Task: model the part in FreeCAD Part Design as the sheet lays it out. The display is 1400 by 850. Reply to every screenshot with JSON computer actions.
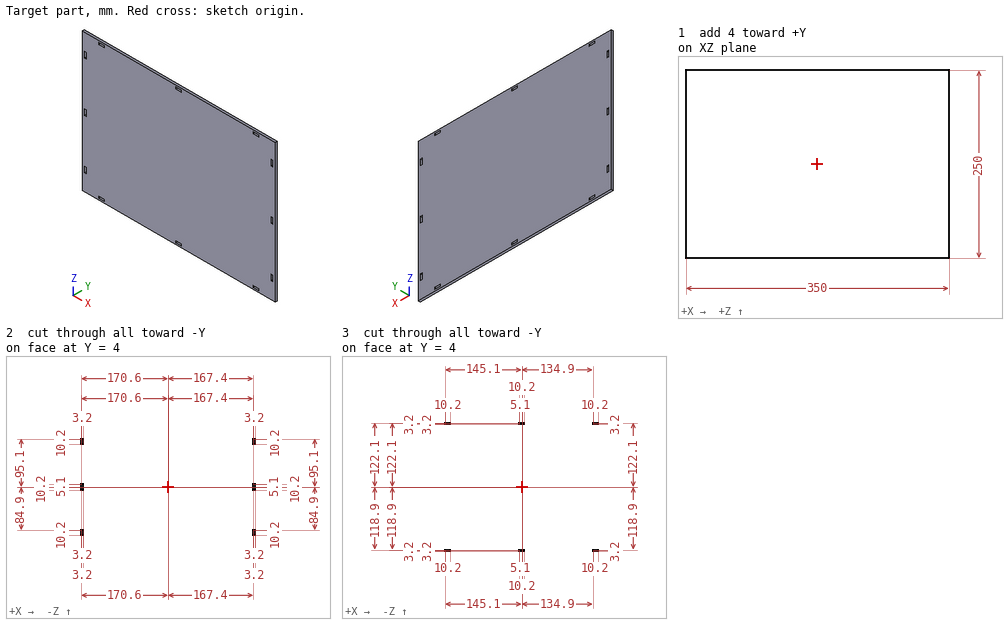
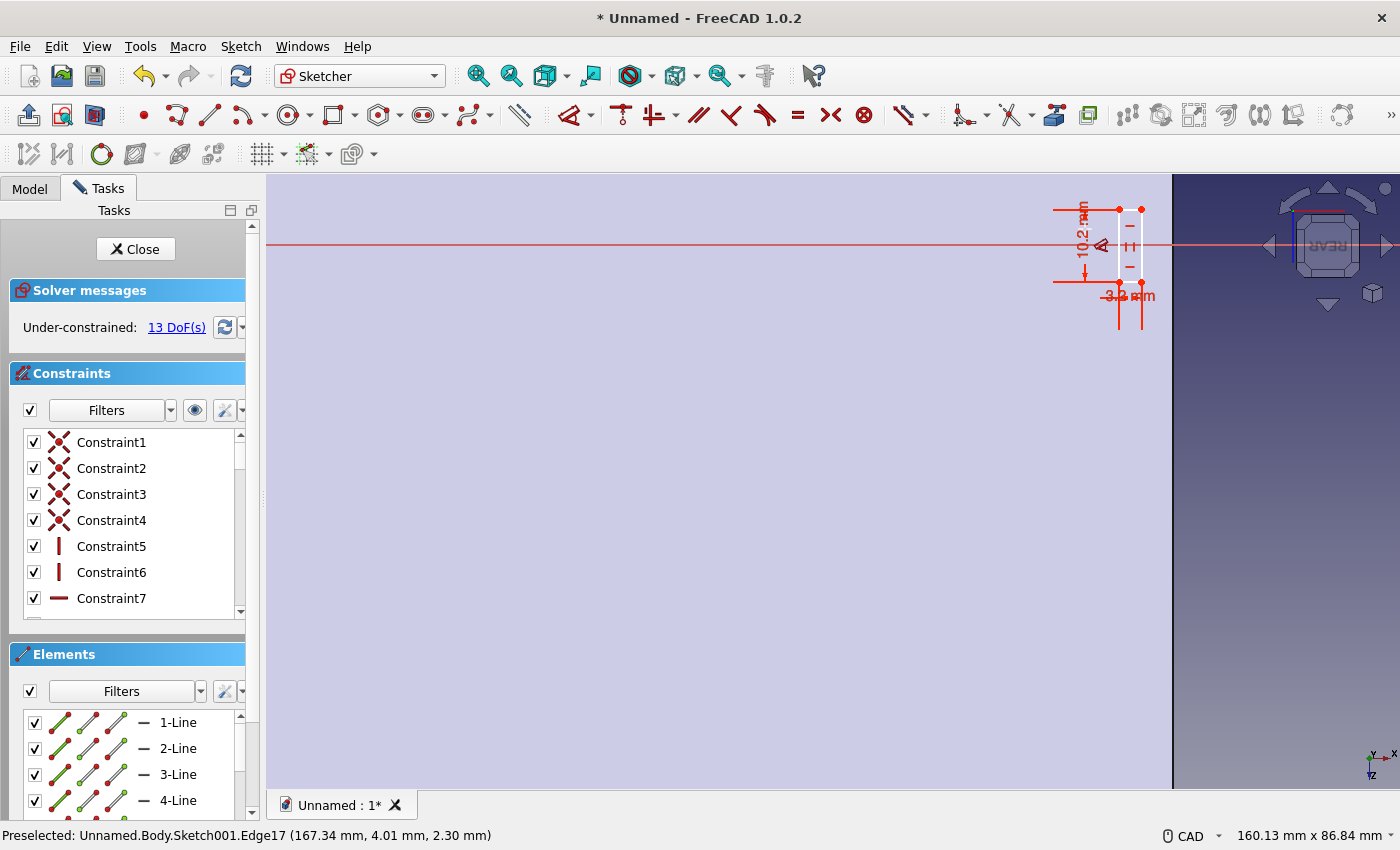
{"action": "scroll", "coordinate": [1122, 584], "scroll_direction": "down", "scroll_amount": 6}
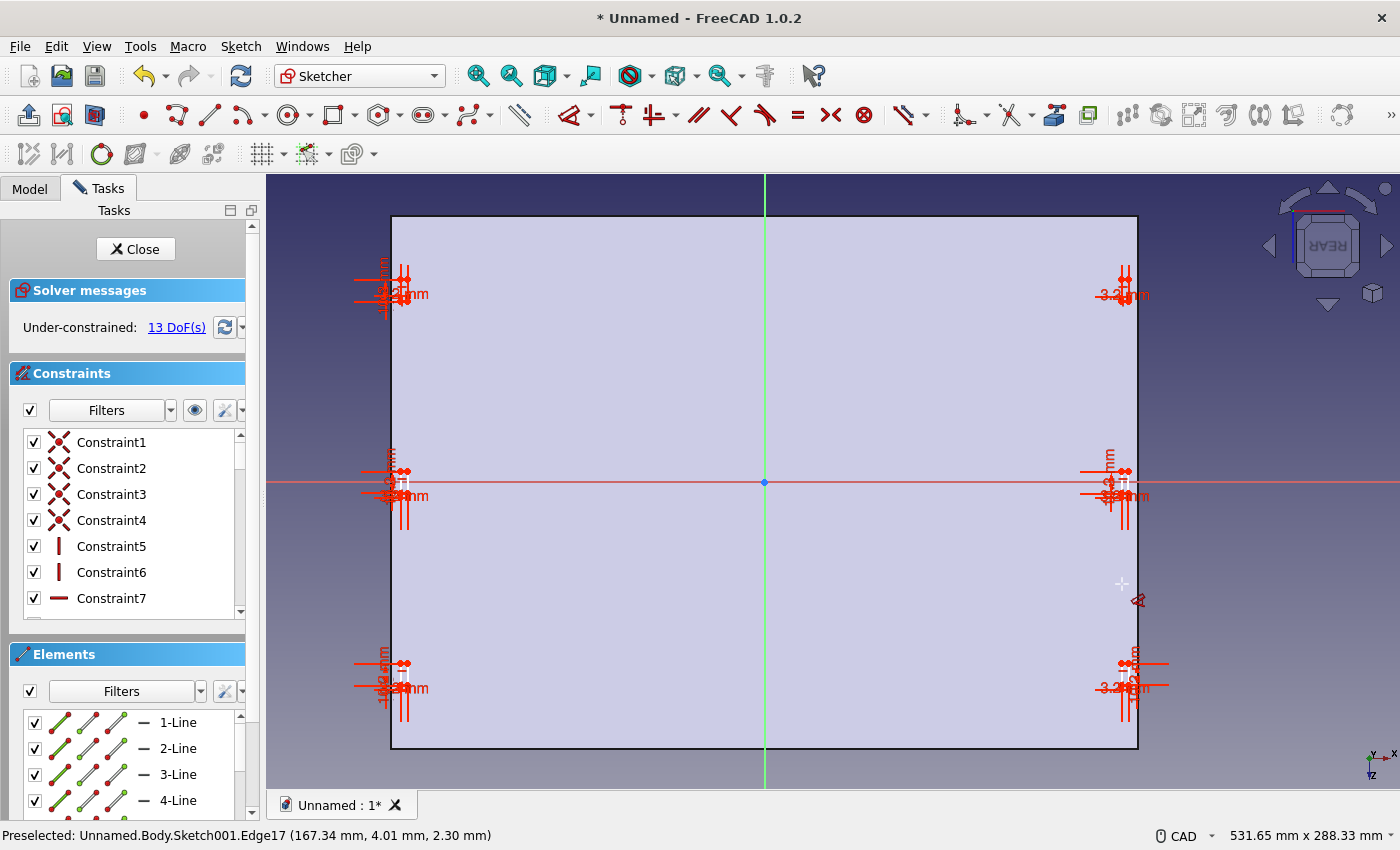
{"action": "scroll", "coordinate": [1122, 286], "scroll_direction": "up", "scroll_amount": 4}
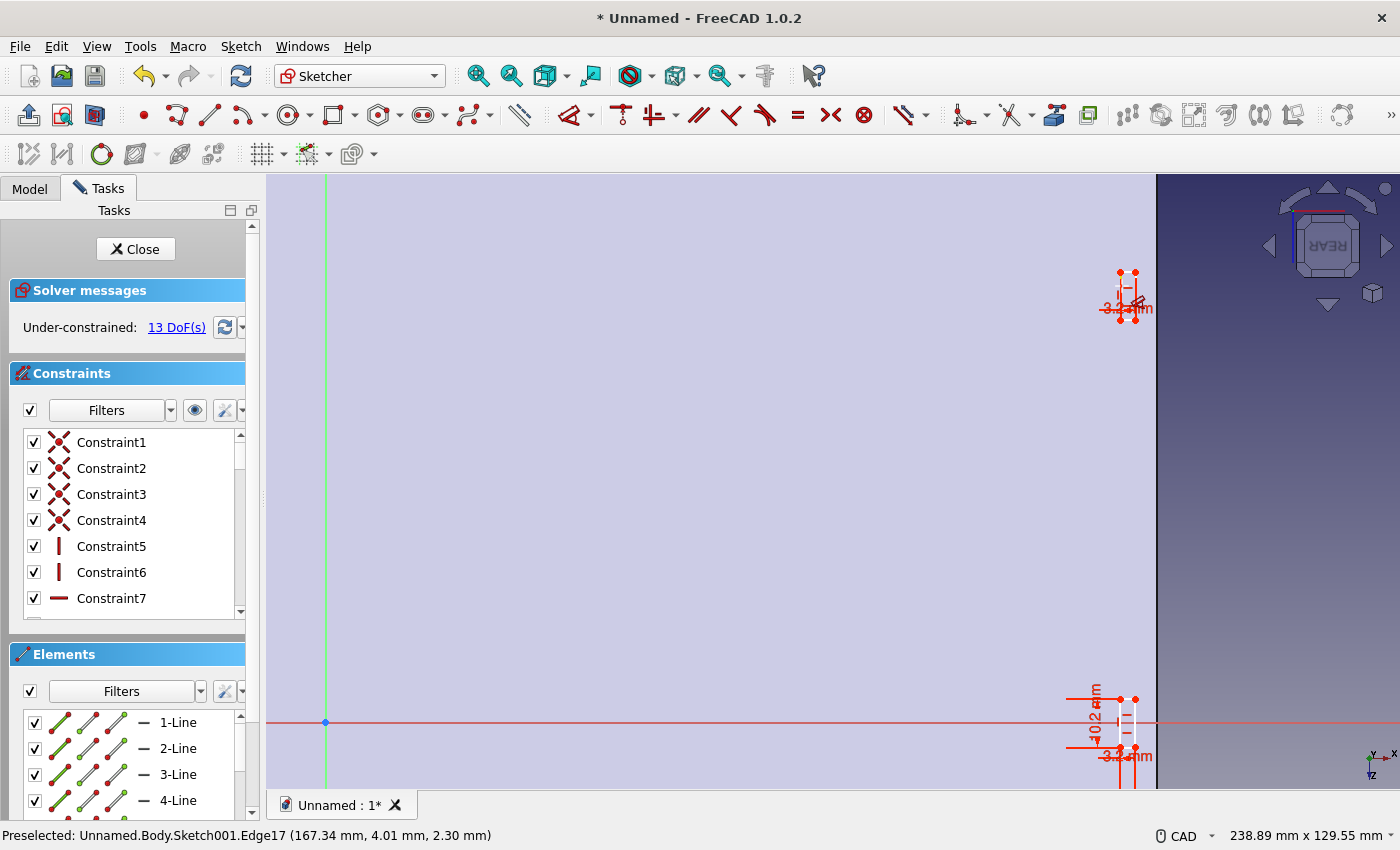
{"action": "left_click", "coordinate": [1121, 287]}
{"action": "left_click", "coordinate": [1155, 285]}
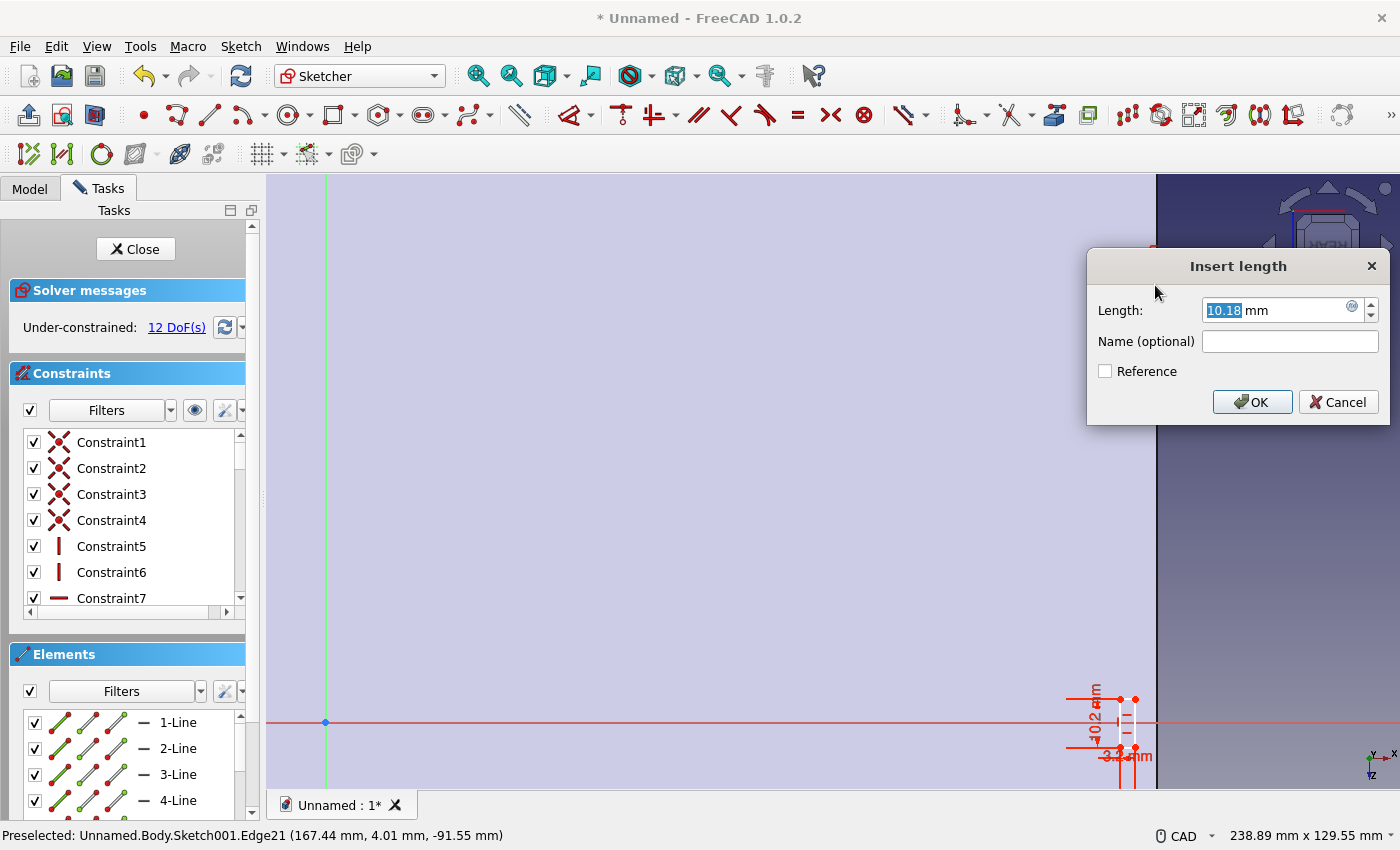
{"action": "type", "text": "10.2"}
{"action": "key", "text": "Return"}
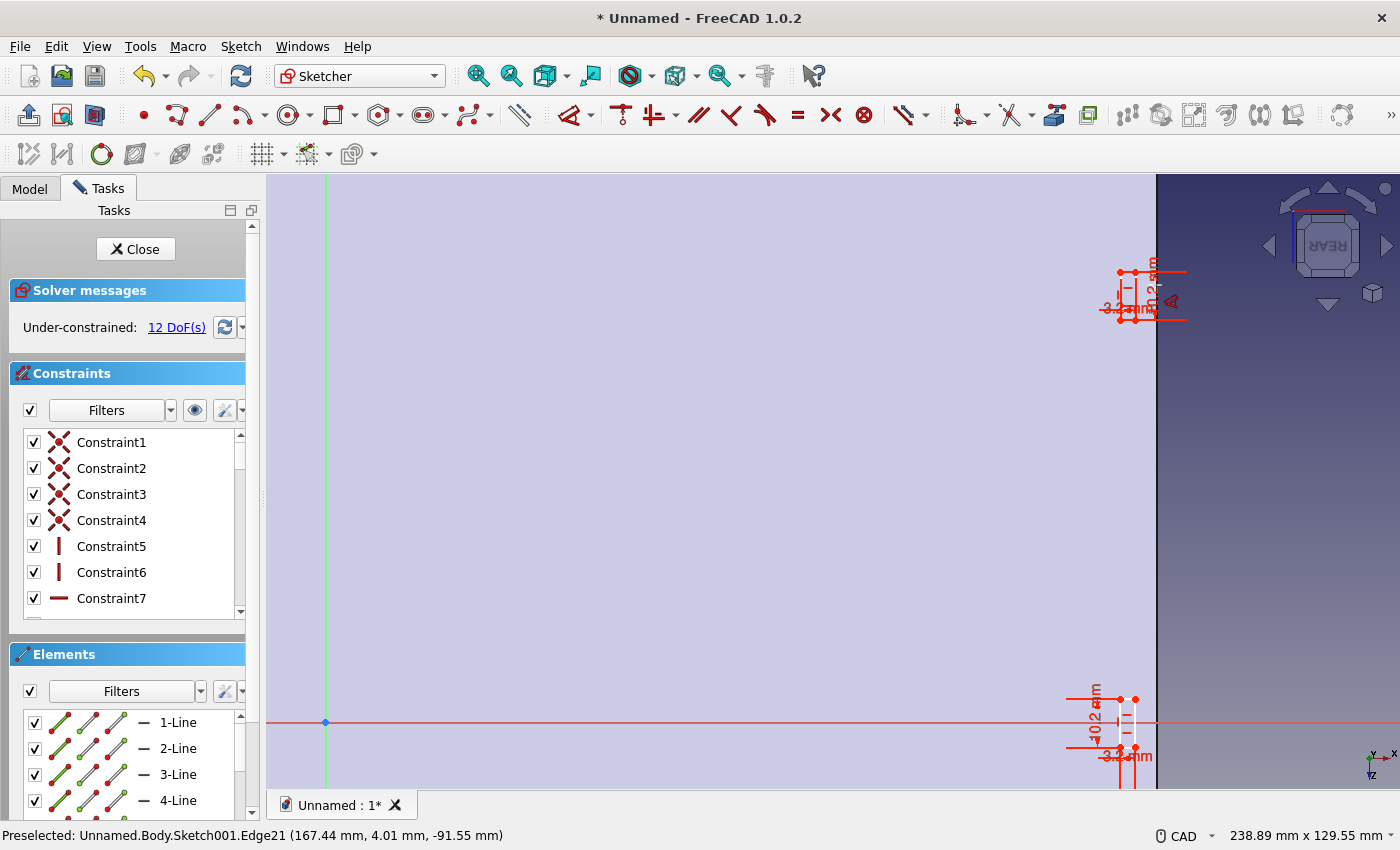
{"action": "scroll", "coordinate": [1122, 285], "scroll_direction": "down", "scroll_amount": 4}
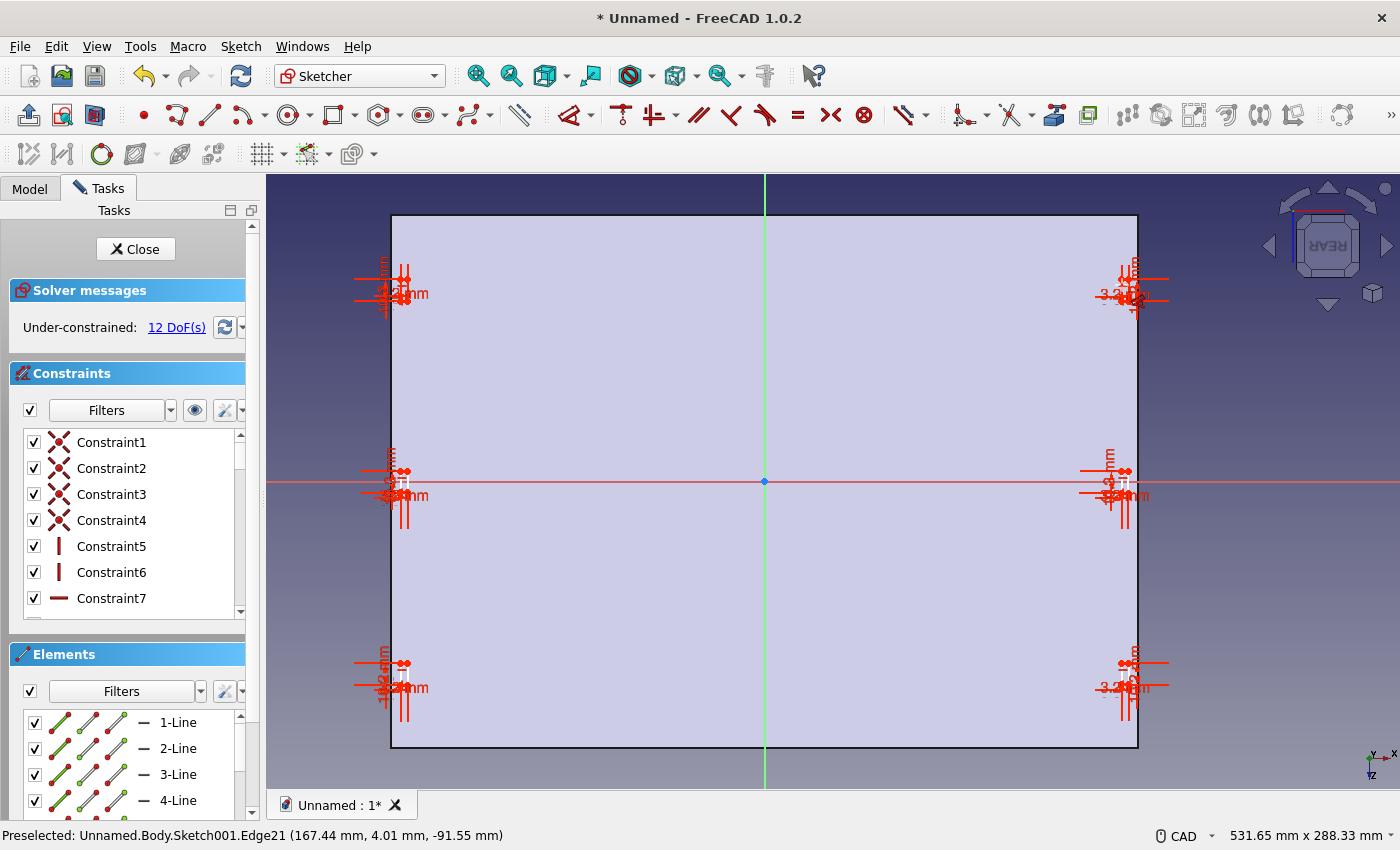
{"action": "scroll", "coordinate": [401, 471], "scroll_direction": "up", "scroll_amount": 7}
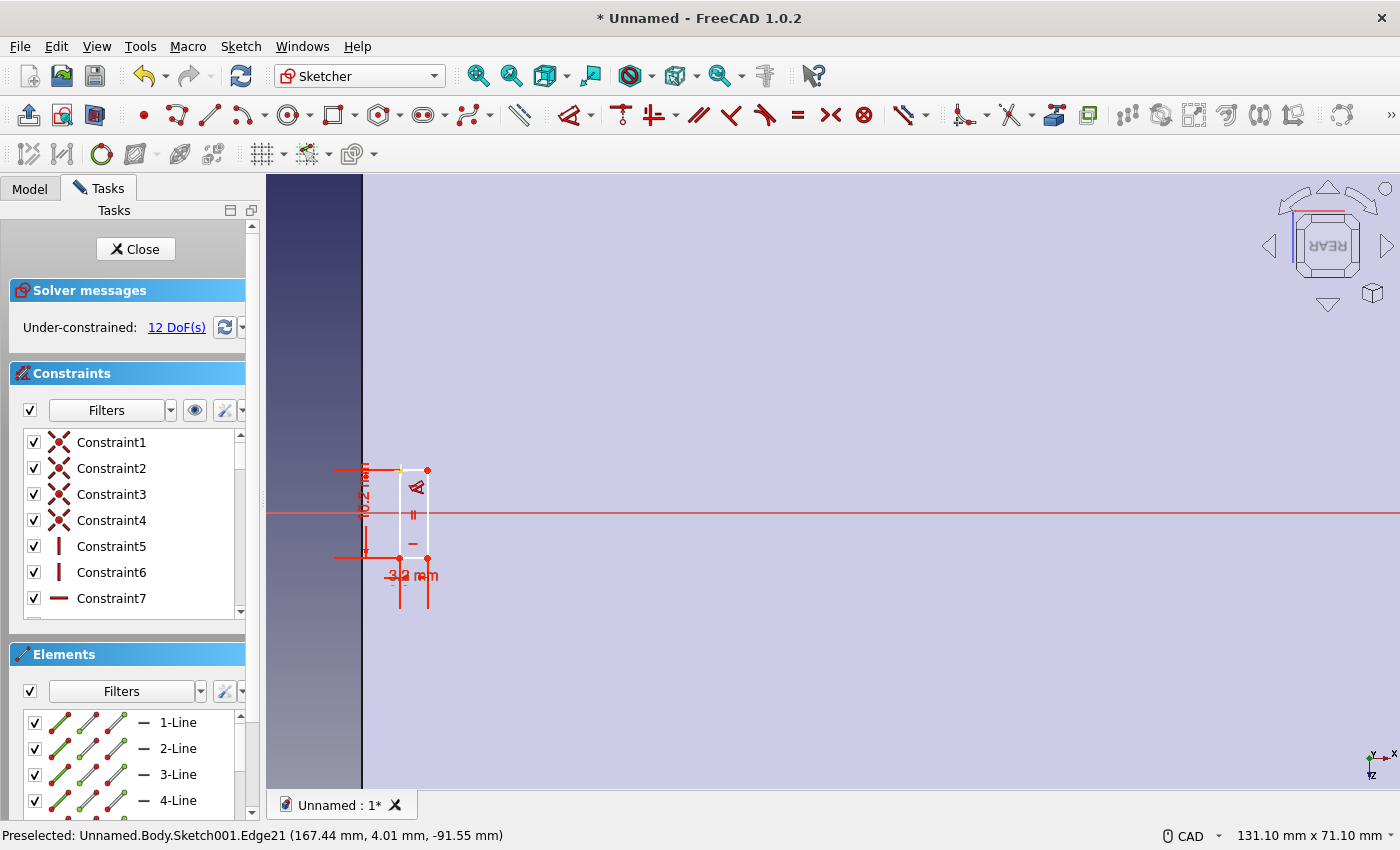
{"action": "left_click", "coordinate": [400, 470]}
{"action": "left_click", "coordinate": [366, 501]}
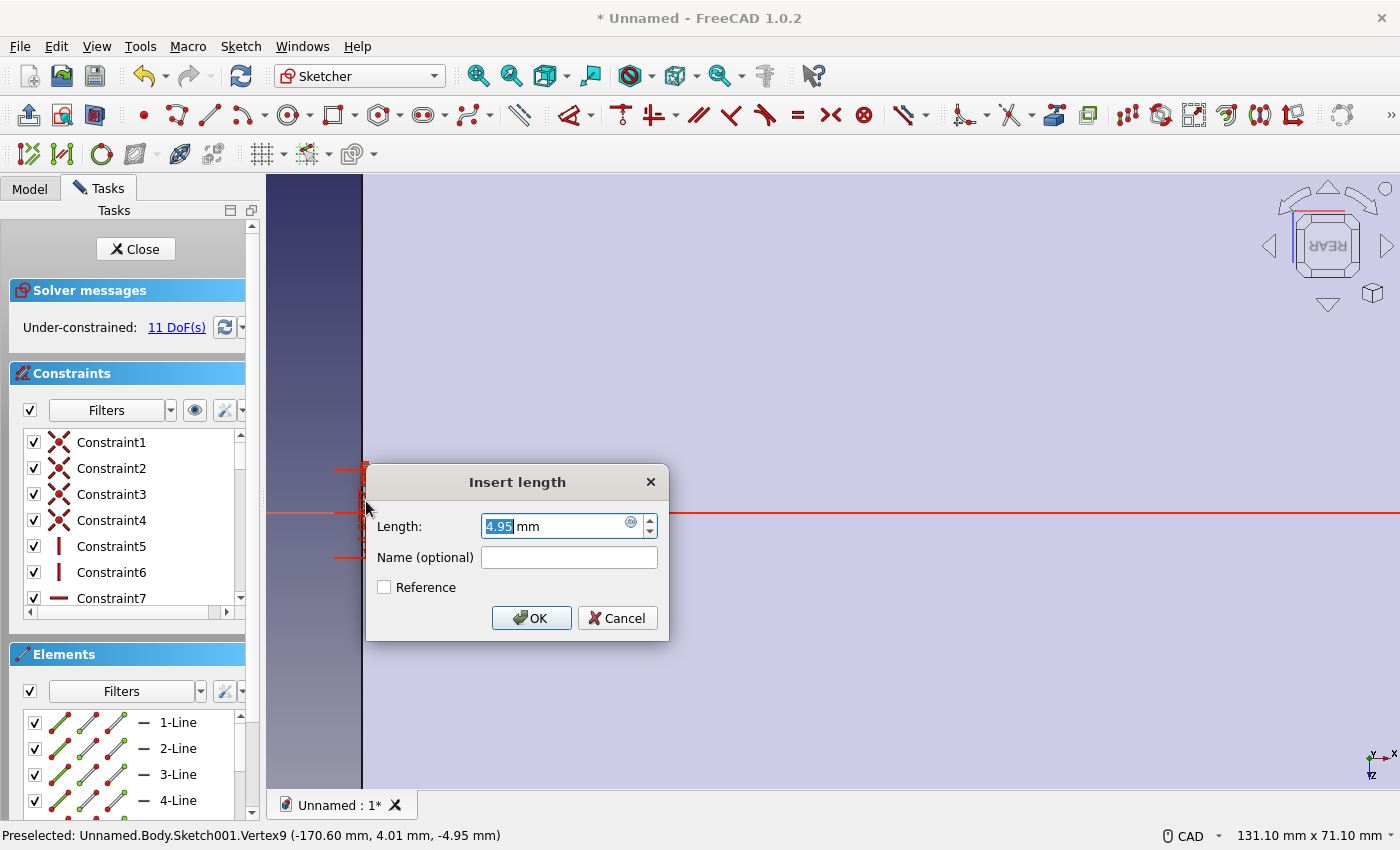
{"action": "type", "text": "5.1"}
{"action": "key", "text": "Return"}